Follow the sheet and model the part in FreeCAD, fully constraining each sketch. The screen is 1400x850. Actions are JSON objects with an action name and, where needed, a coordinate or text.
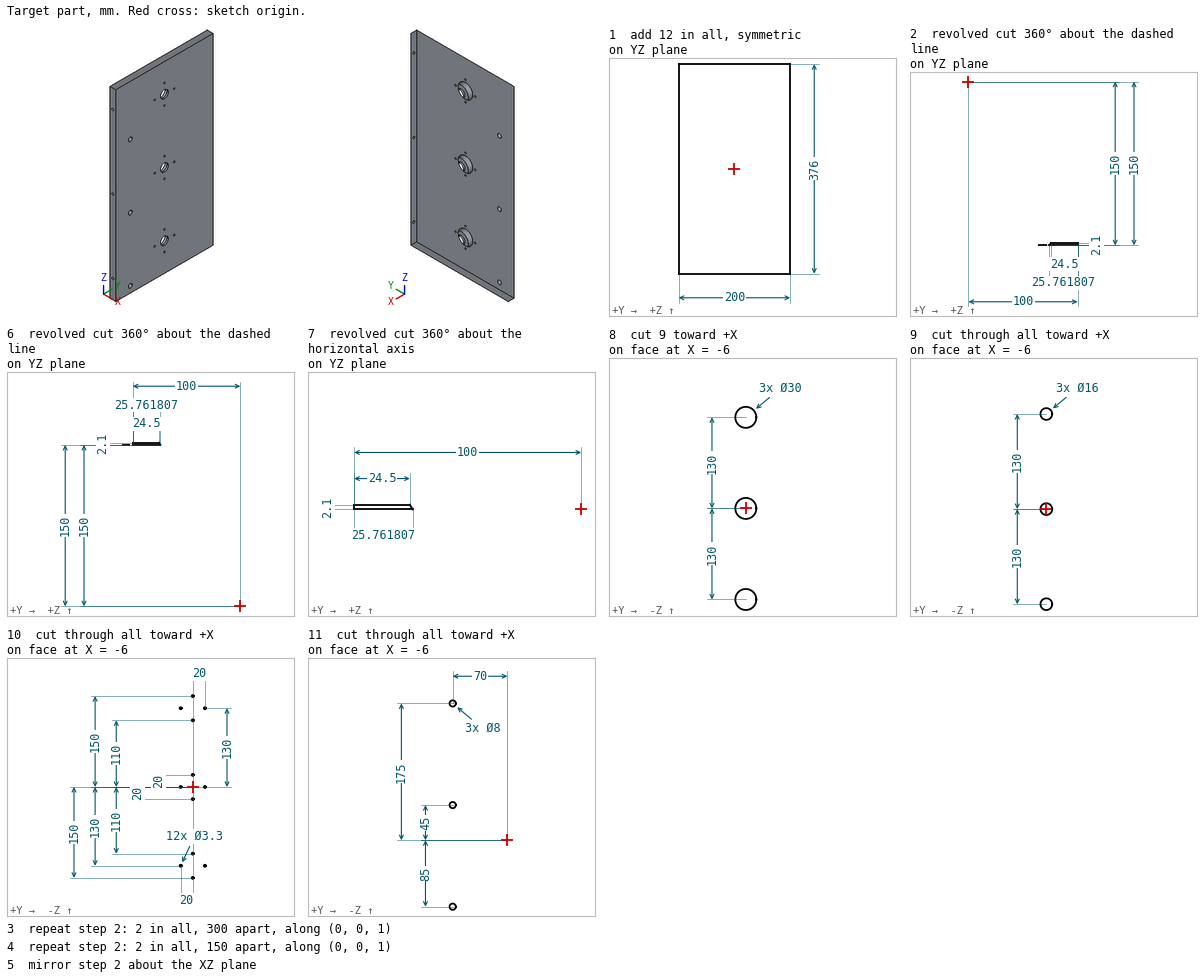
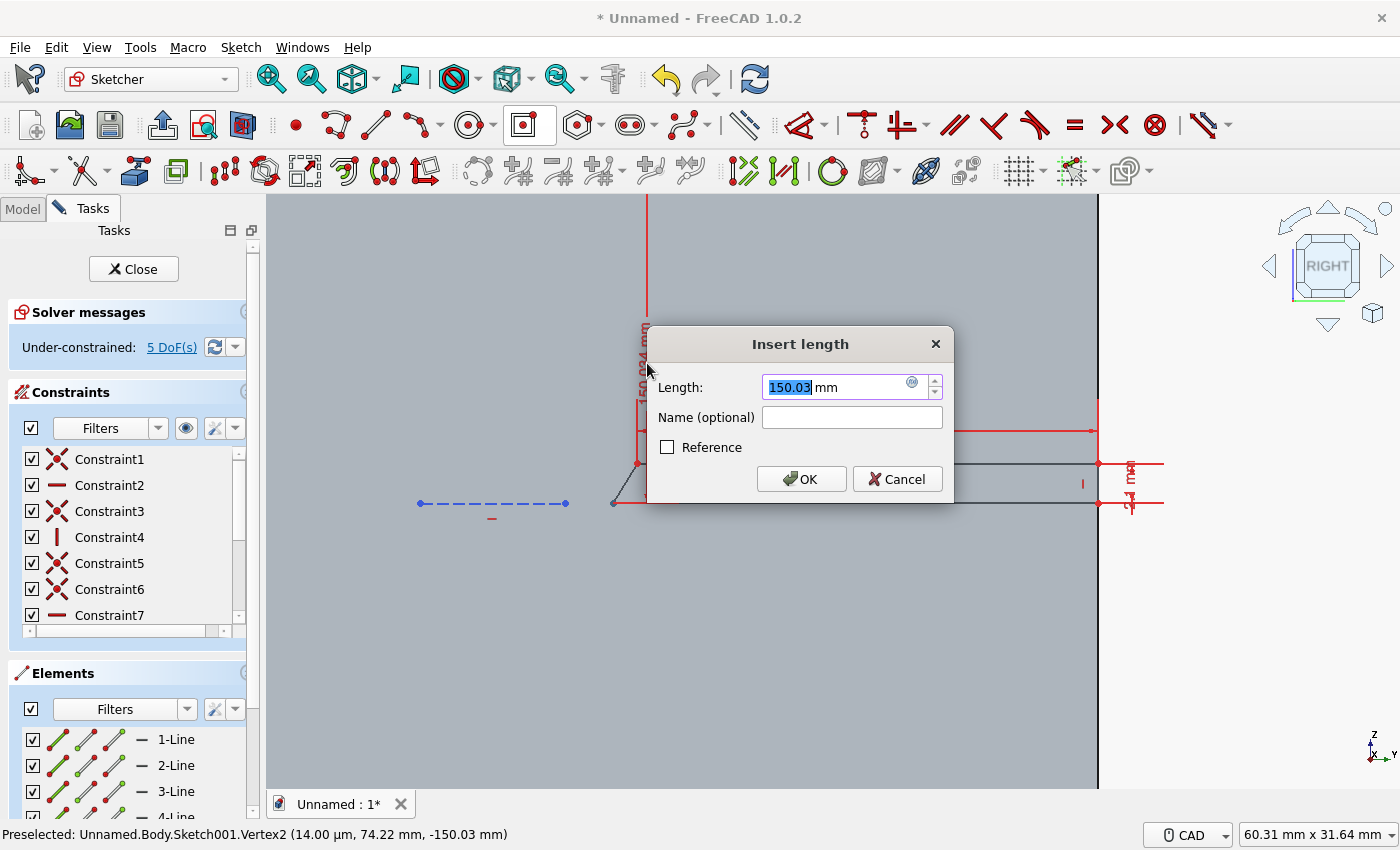
{"action": "type", "text": "150"}
{"action": "key", "text": "Return"}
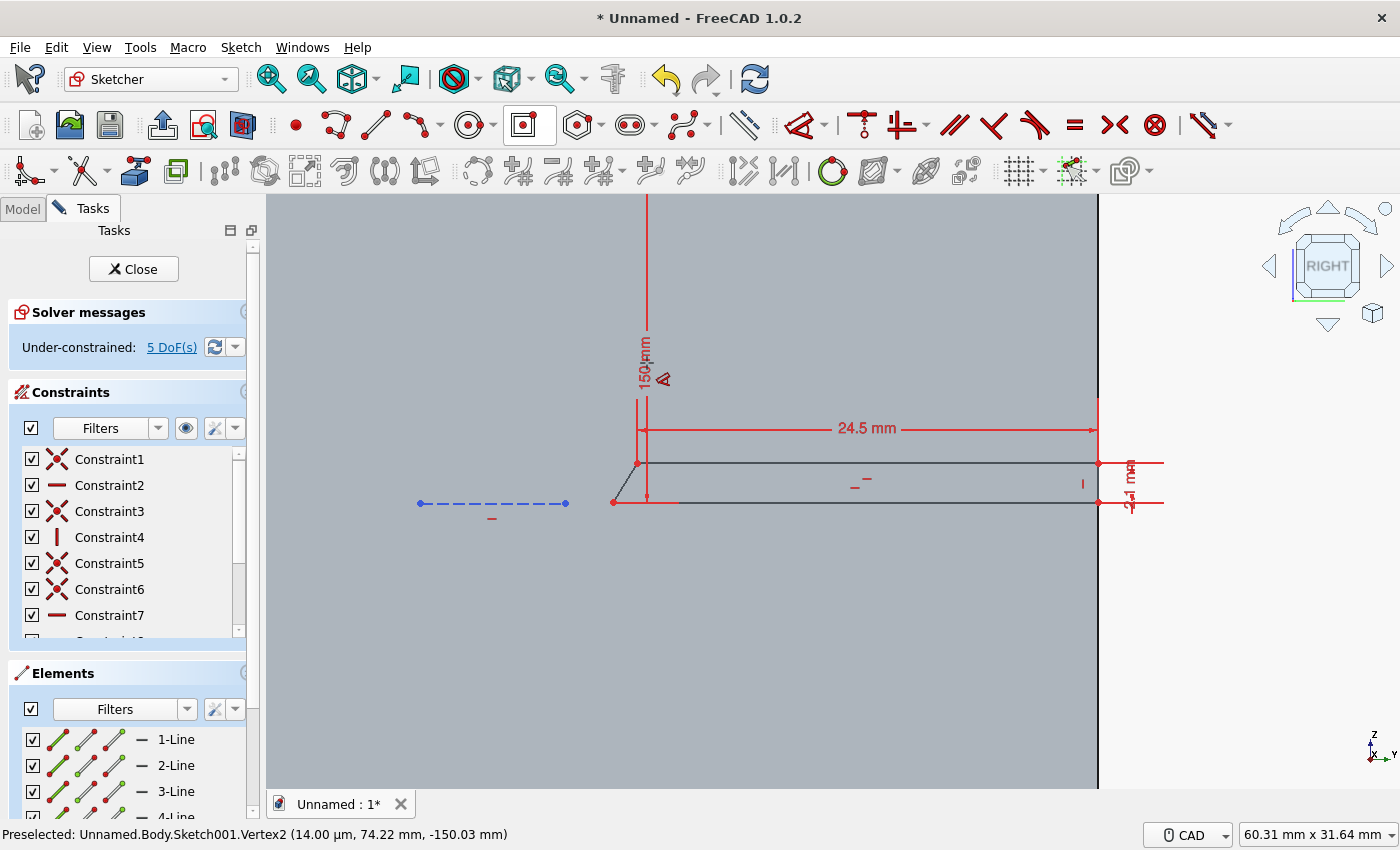
{"action": "left_click", "coordinate": [1098, 503]}
{"action": "left_click", "coordinate": [696, 537]}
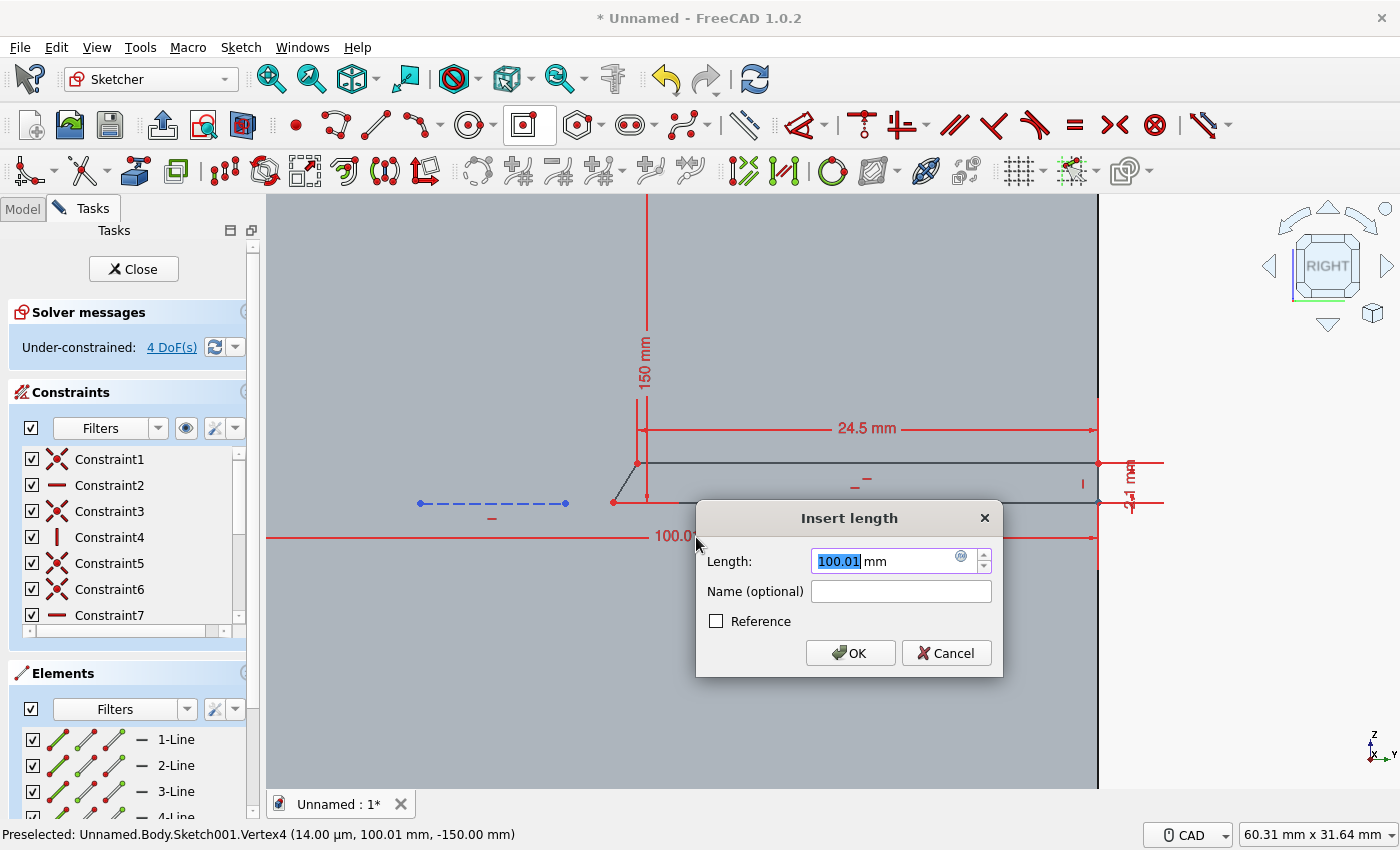
{"action": "type", "text": "100"}
{"action": "key", "text": "Return"}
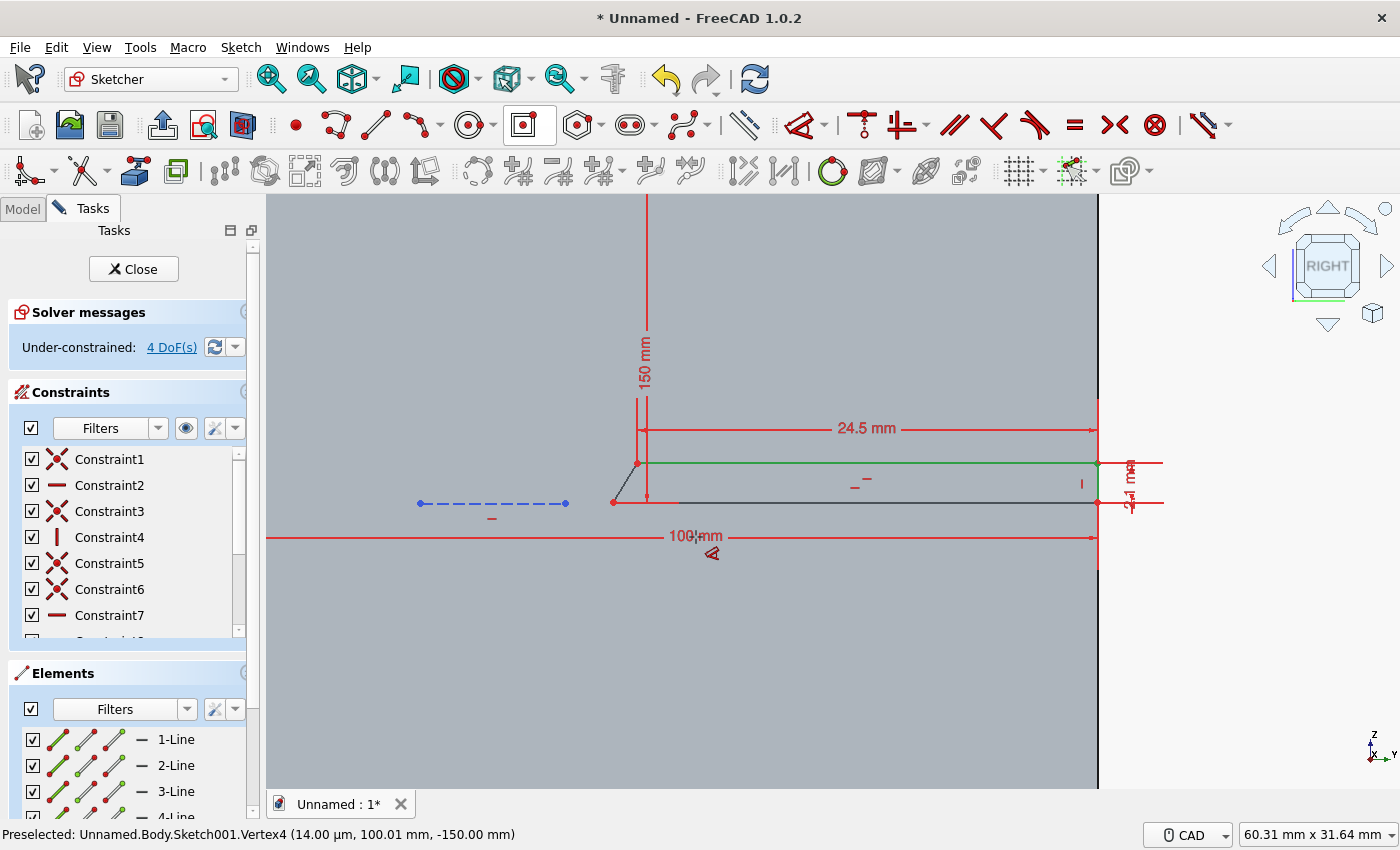
{"action": "left_click", "coordinate": [565, 504]}
{"action": "left_click", "coordinate": [599, 298]}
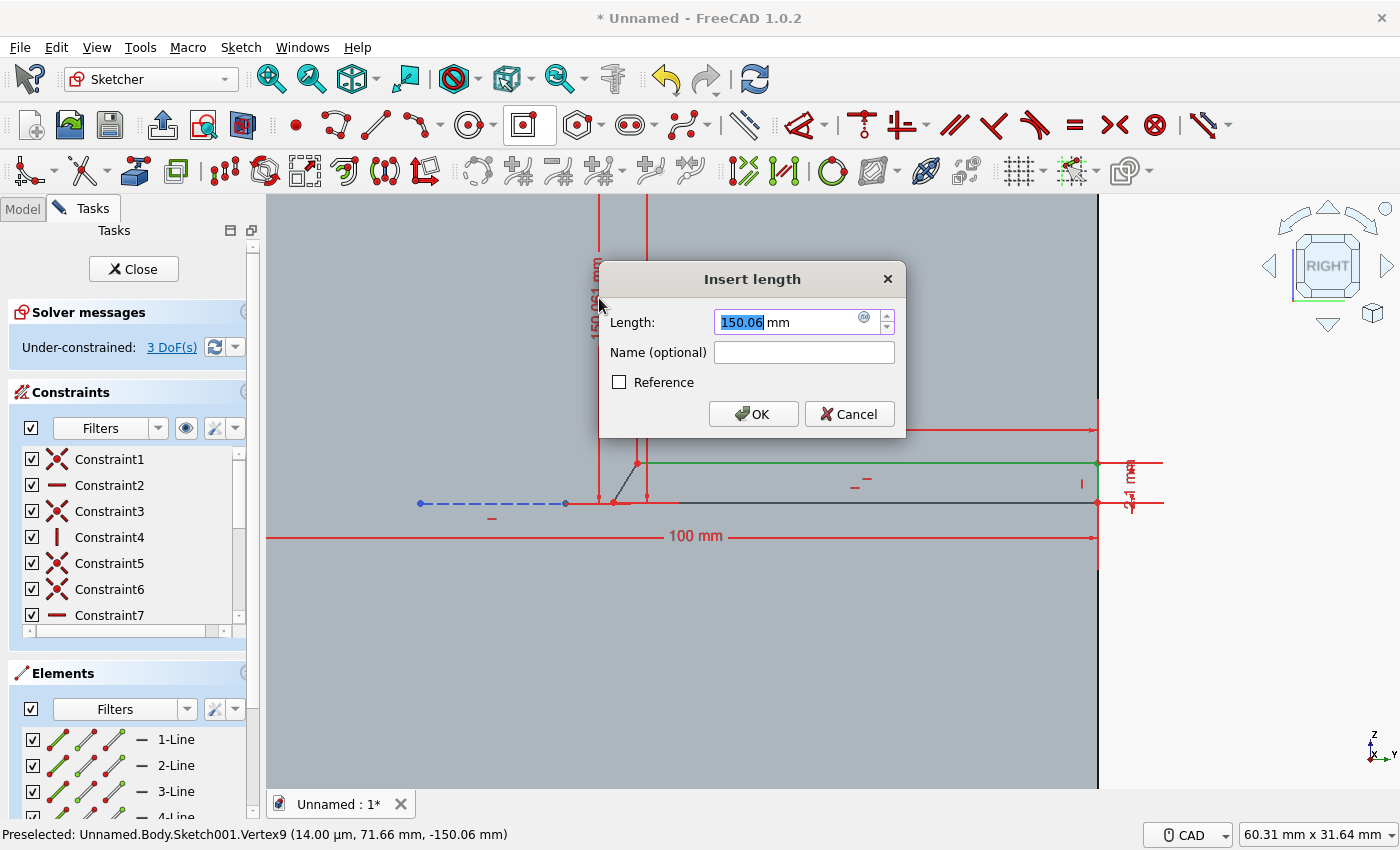
{"action": "type", "text": "150"}
{"action": "key", "text": "Return"}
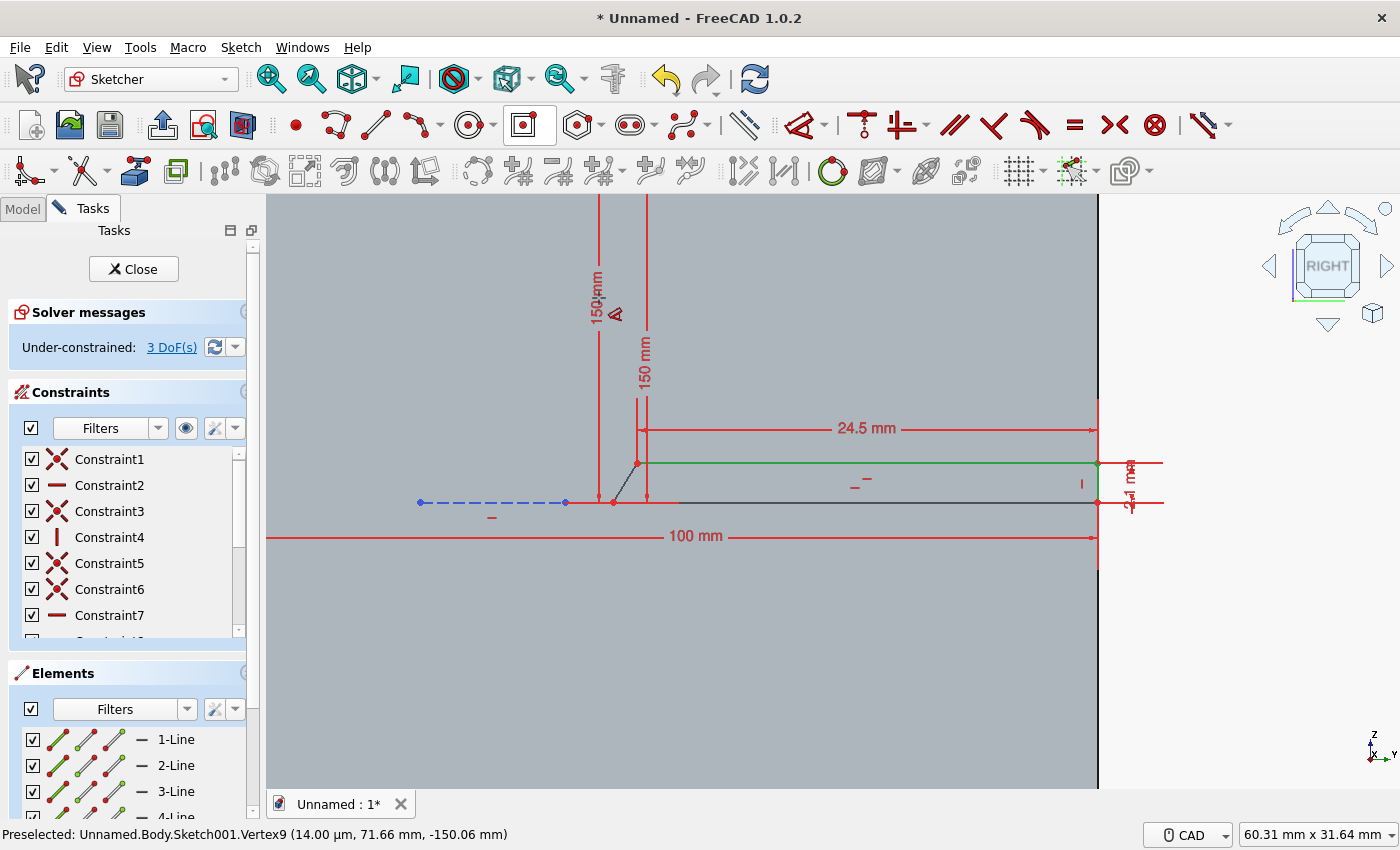
{"action": "left_click", "coordinate": [758, 503]}
{"action": "left_click", "coordinate": [855, 537]}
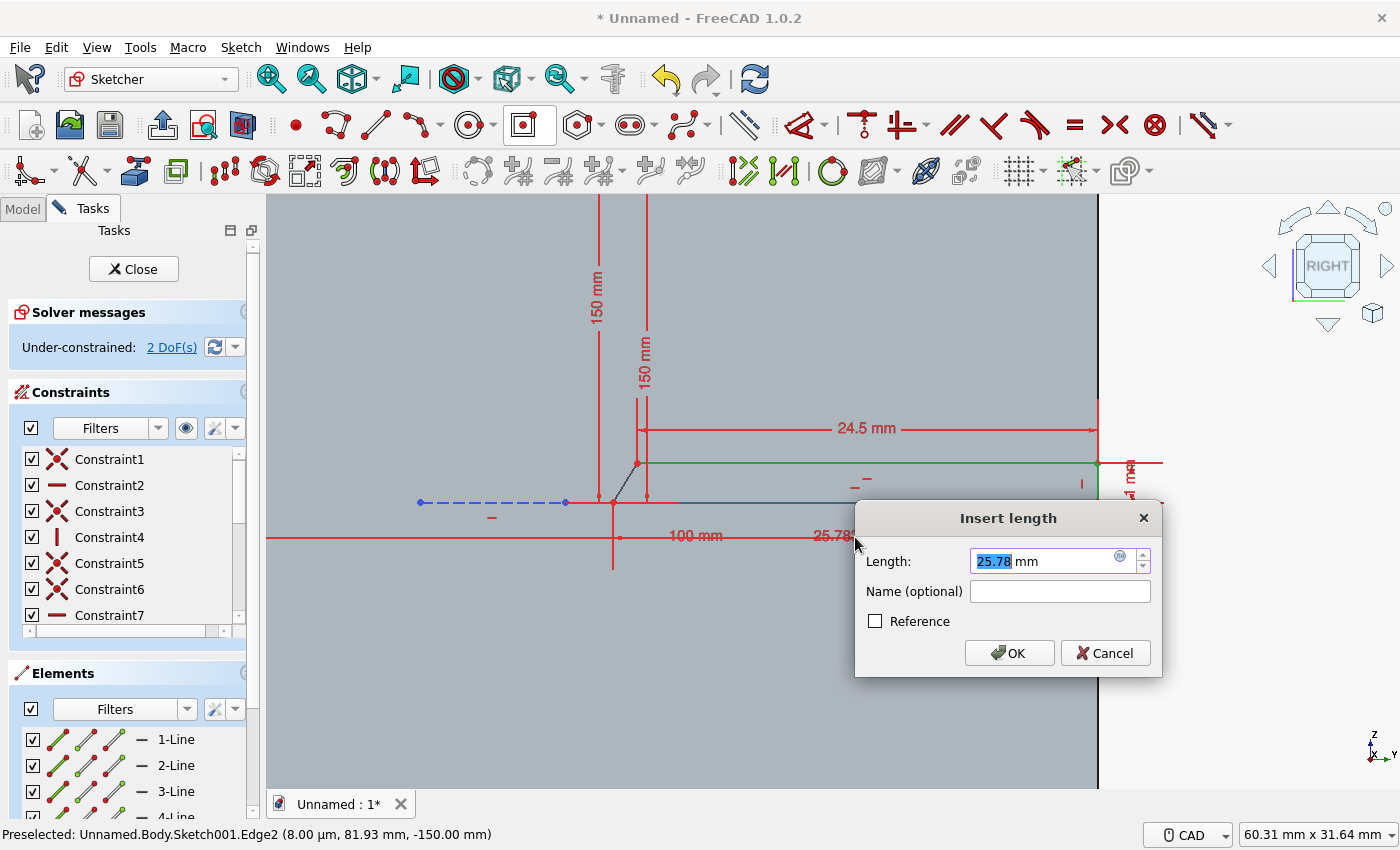
{"action": "type", "text": "25.761807"}
{"action": "key", "text": "Return"}
{"action": "key", "text": "Escape"}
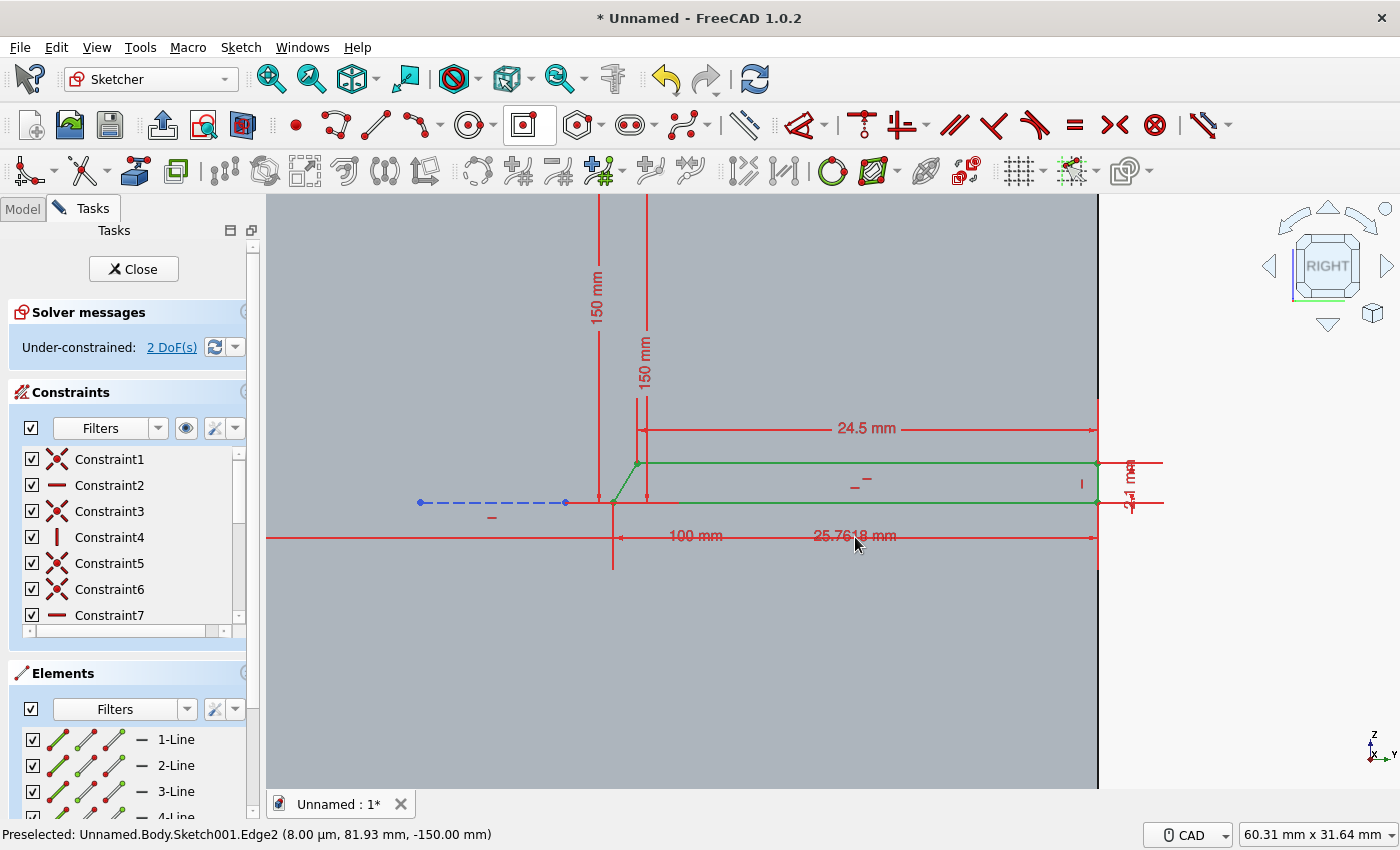
{"action": "left_click", "coordinate": [134, 269]}